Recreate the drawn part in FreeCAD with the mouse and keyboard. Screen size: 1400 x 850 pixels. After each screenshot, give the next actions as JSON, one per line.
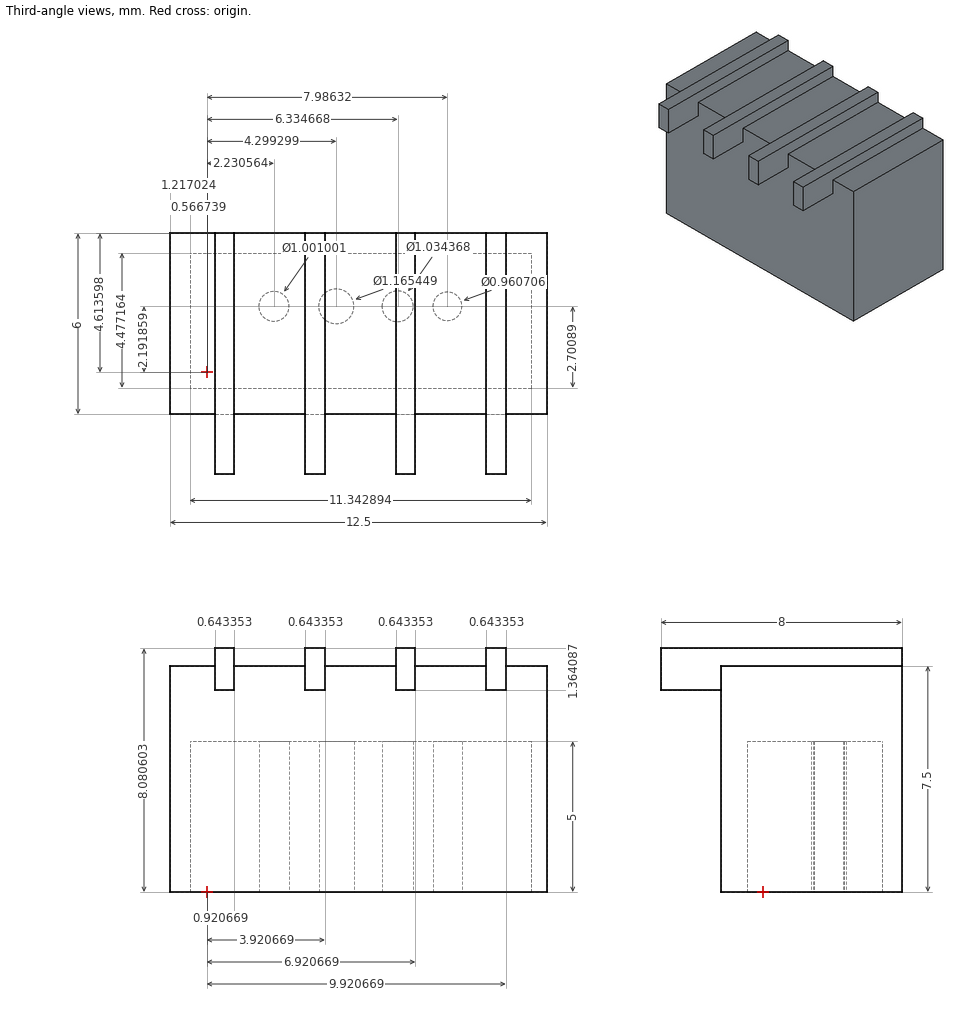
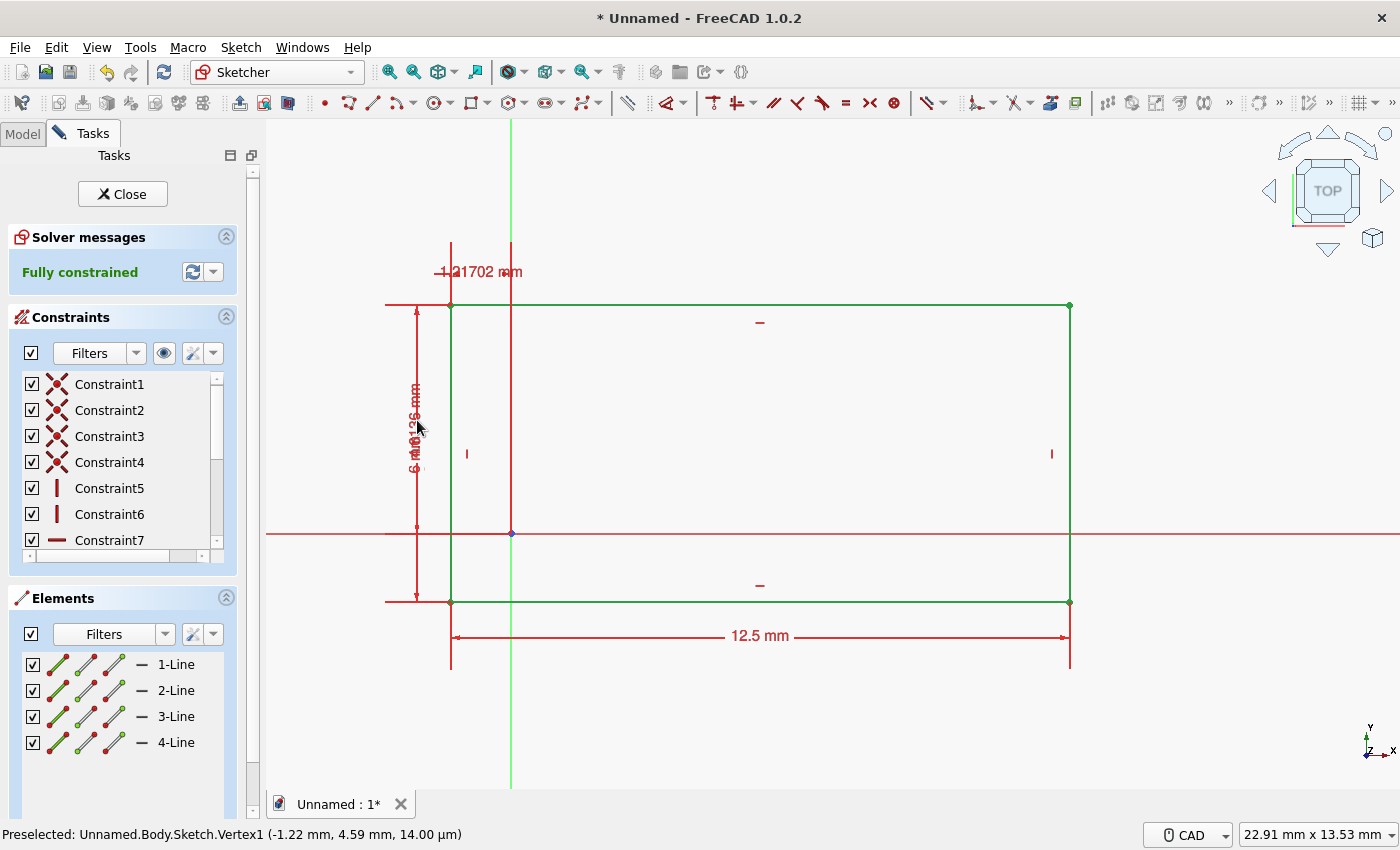
{"action": "left_click", "coordinate": [123, 194]}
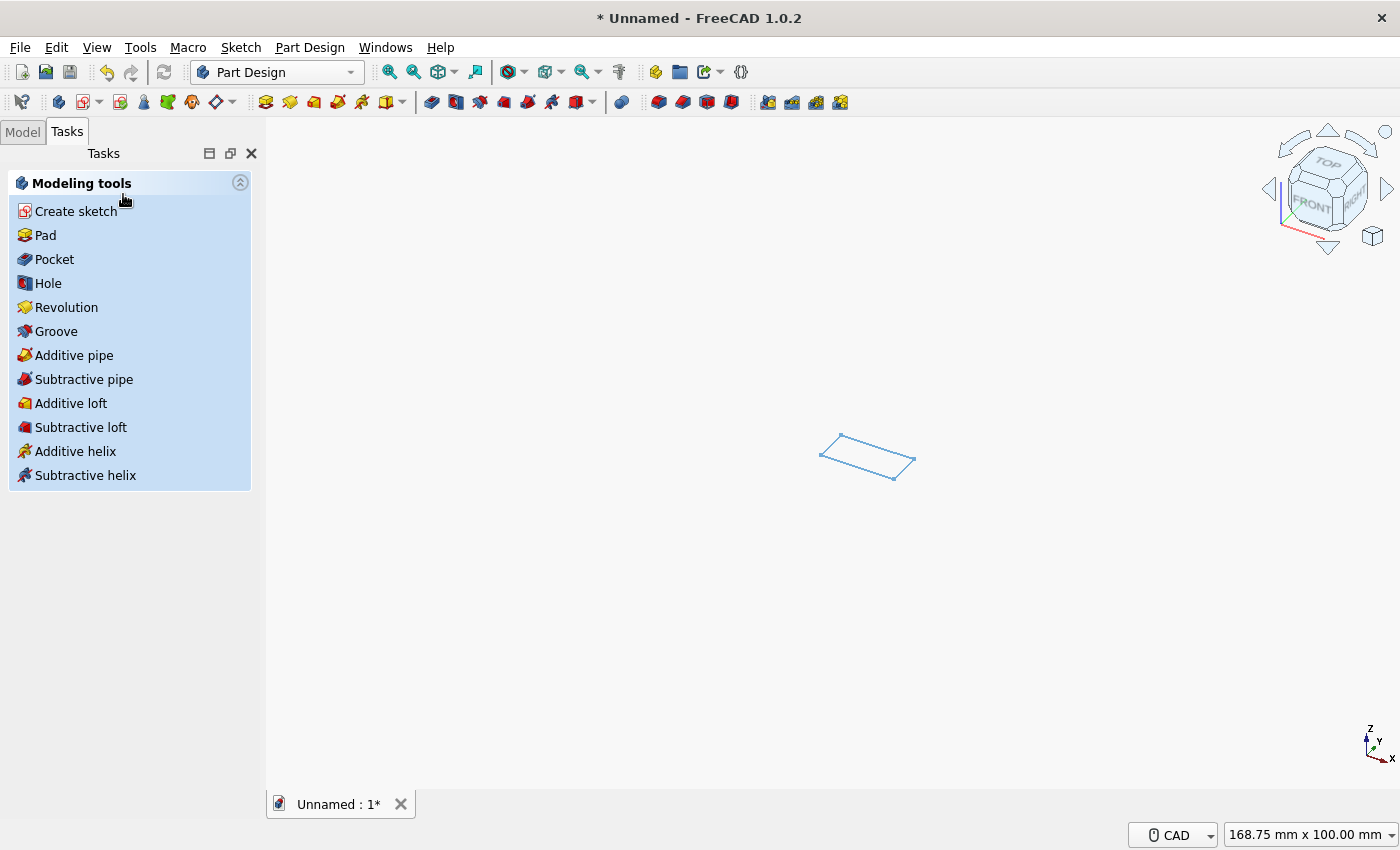
{"action": "left_click", "coordinate": [266, 102]}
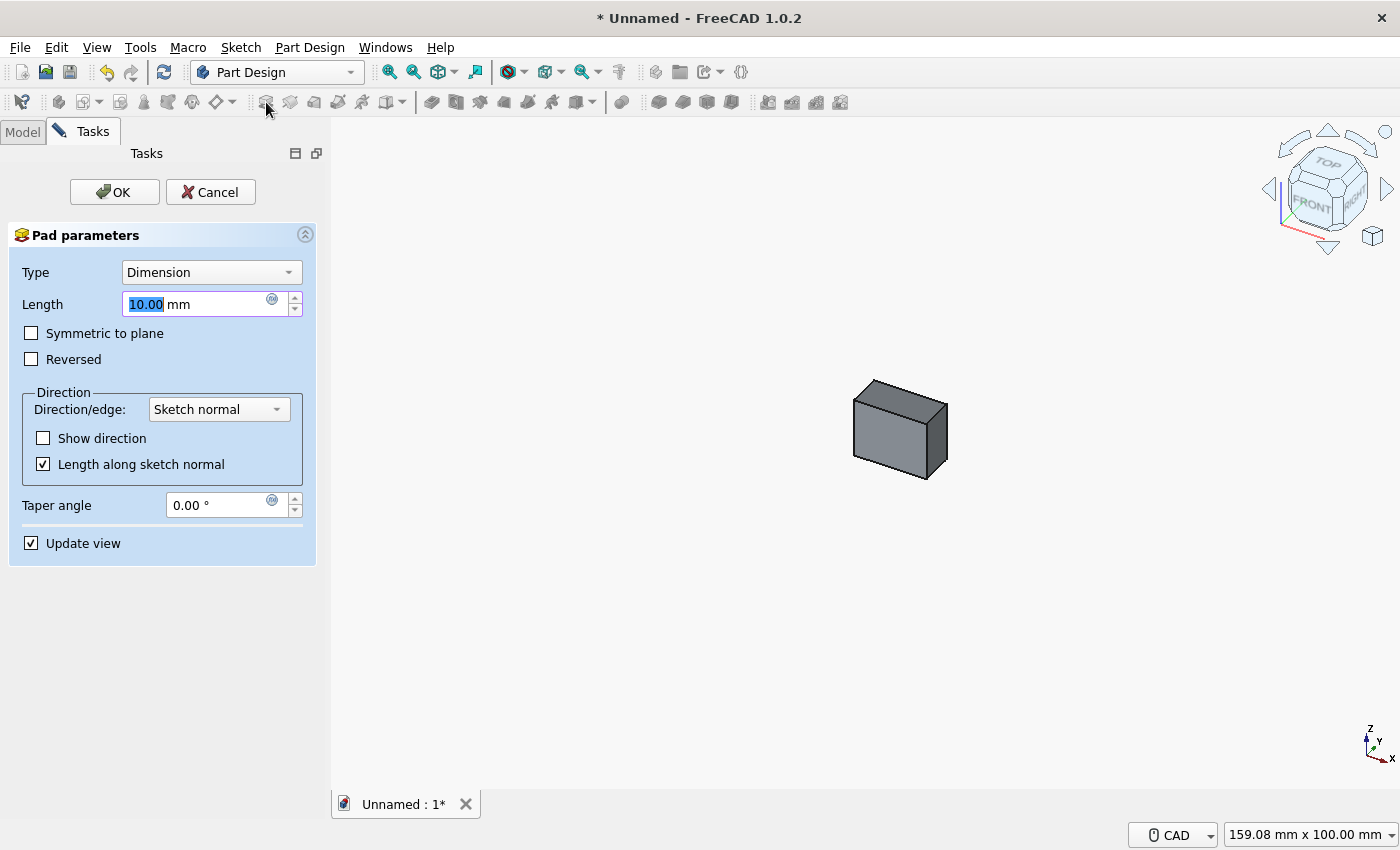
{"action": "type", "text": "7.5"}
{"action": "key", "text": "Tab"}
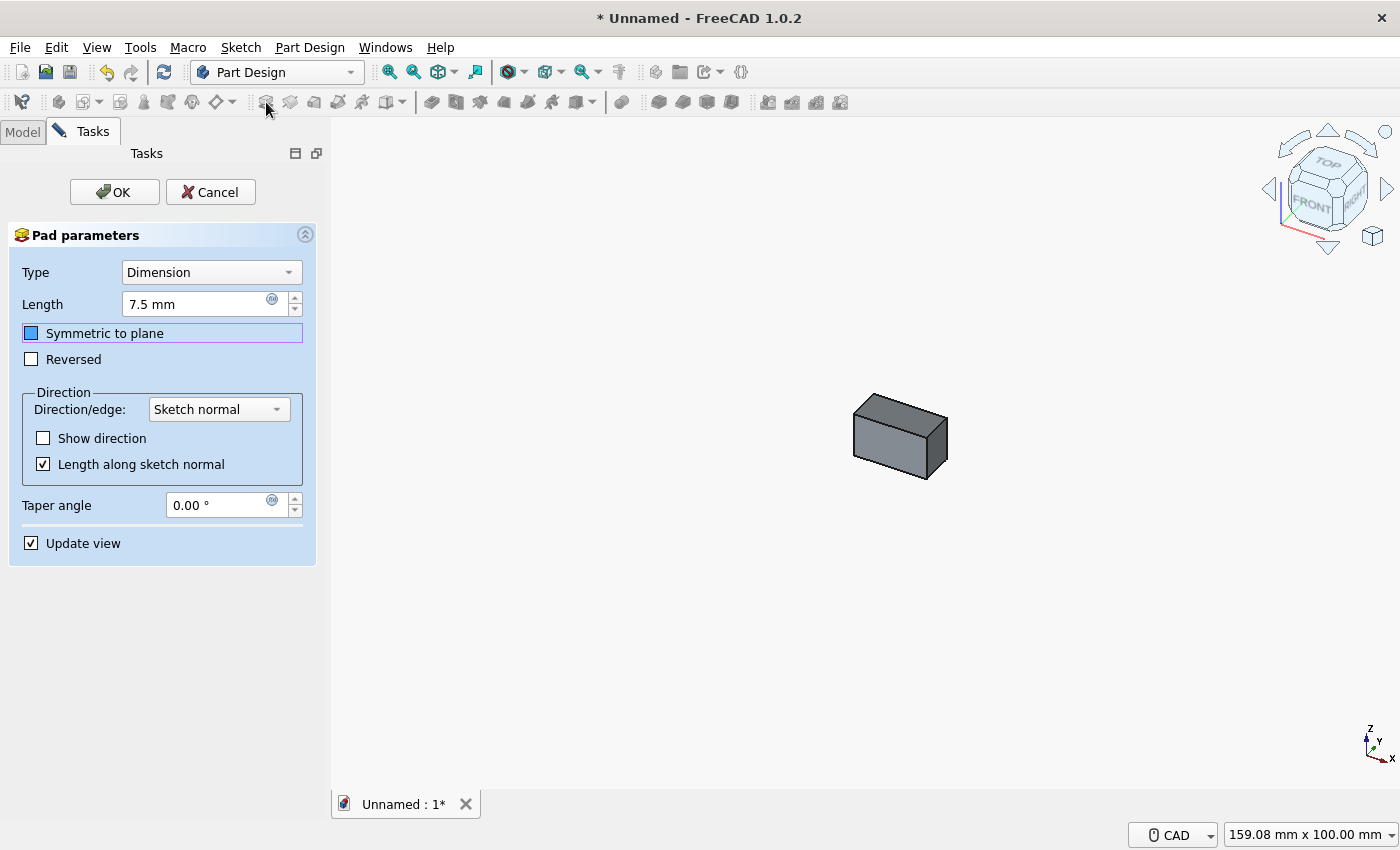
{"action": "left_click", "coordinate": [115, 192]}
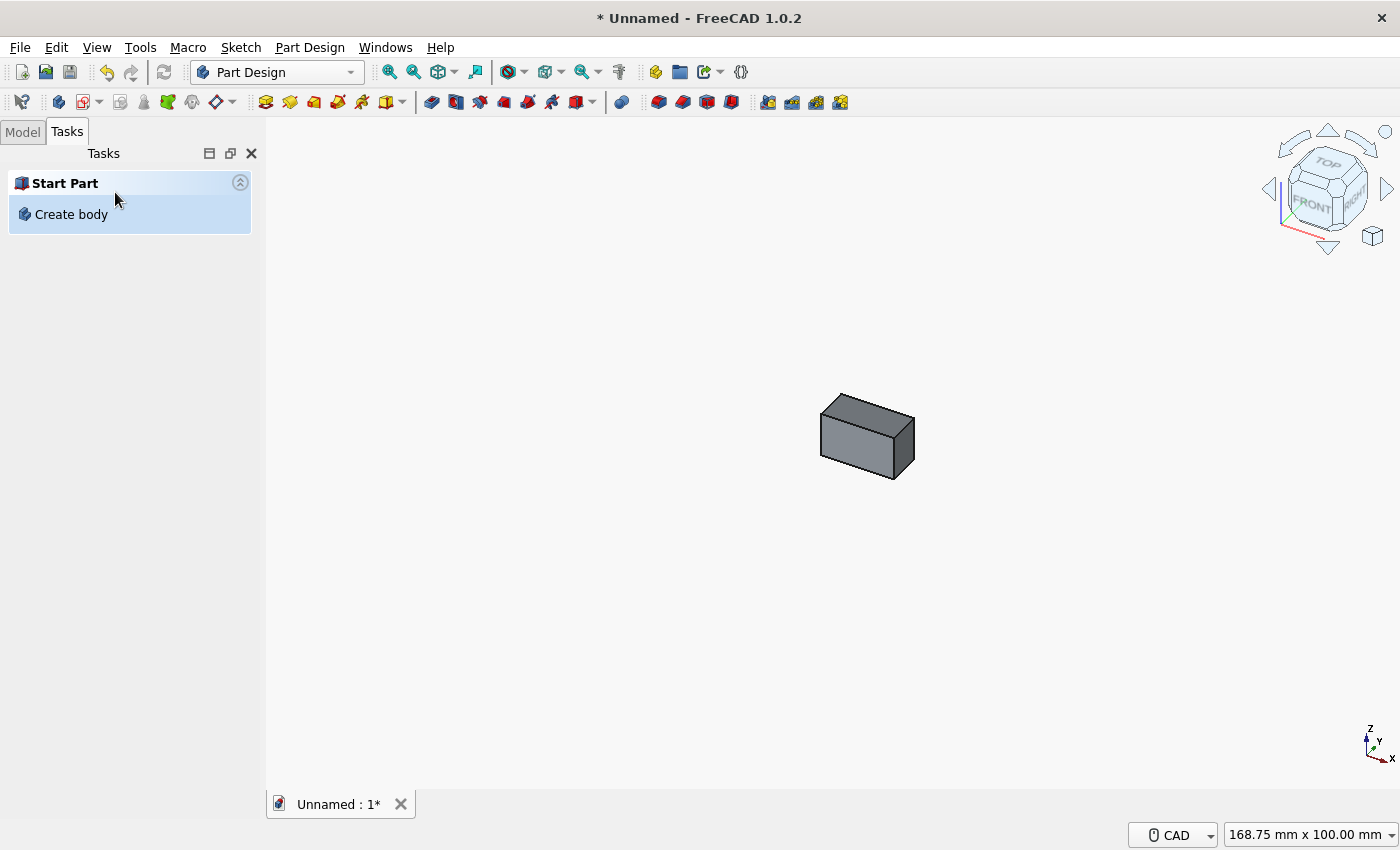
{"action": "key", "text": "v f"}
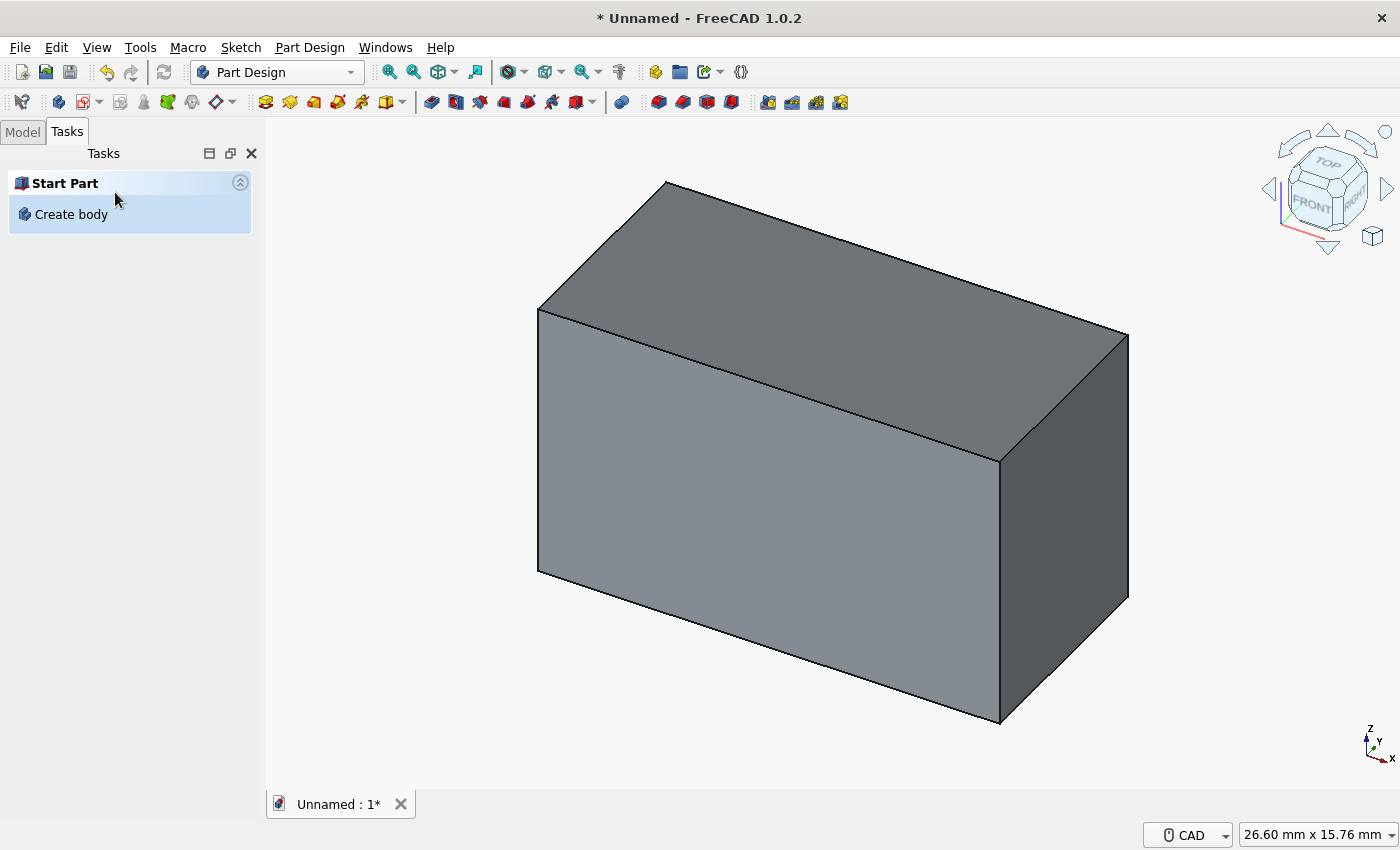
{"action": "left_click", "coordinate": [84, 102]}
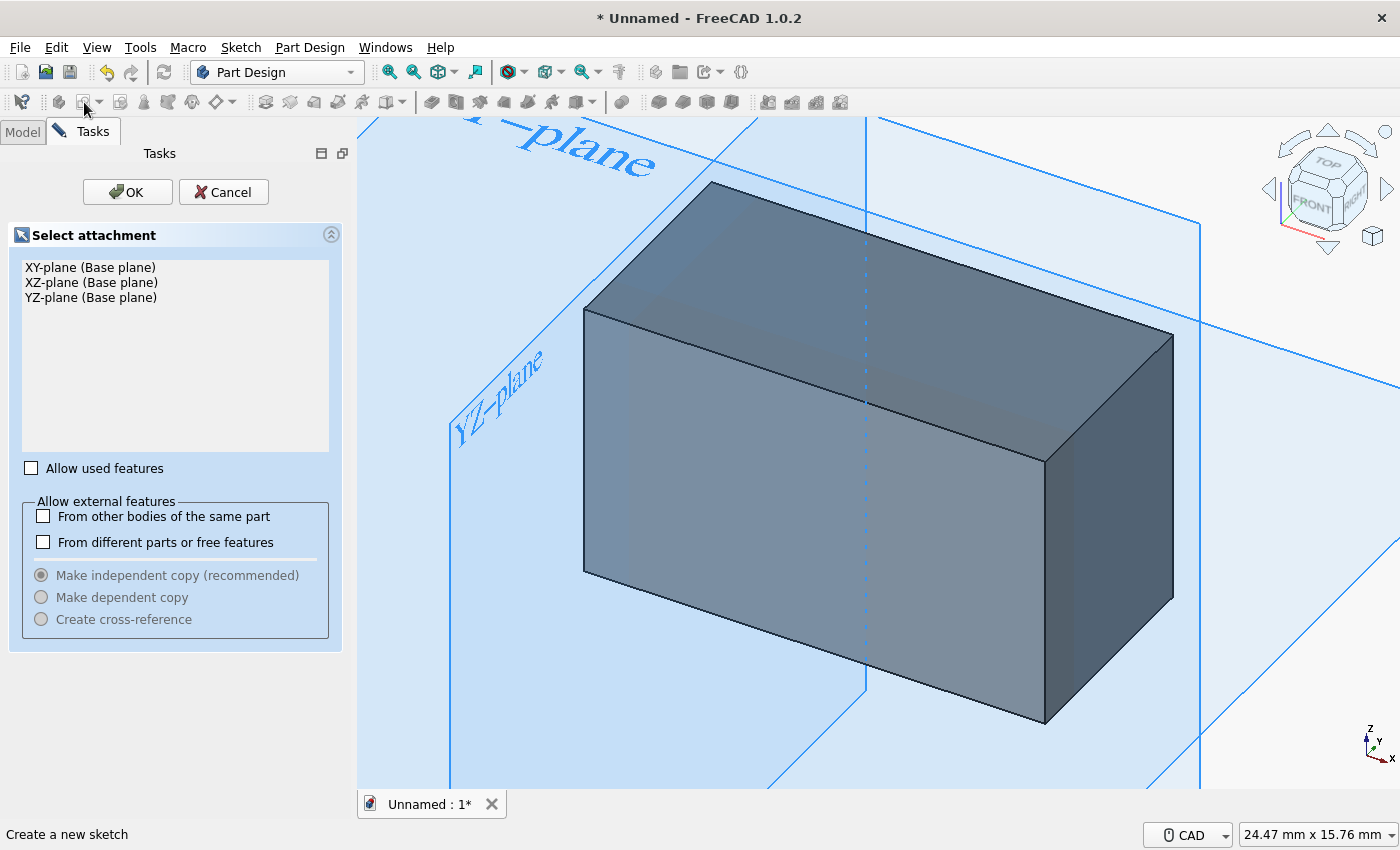
{"action": "left_click", "coordinate": [82, 268]}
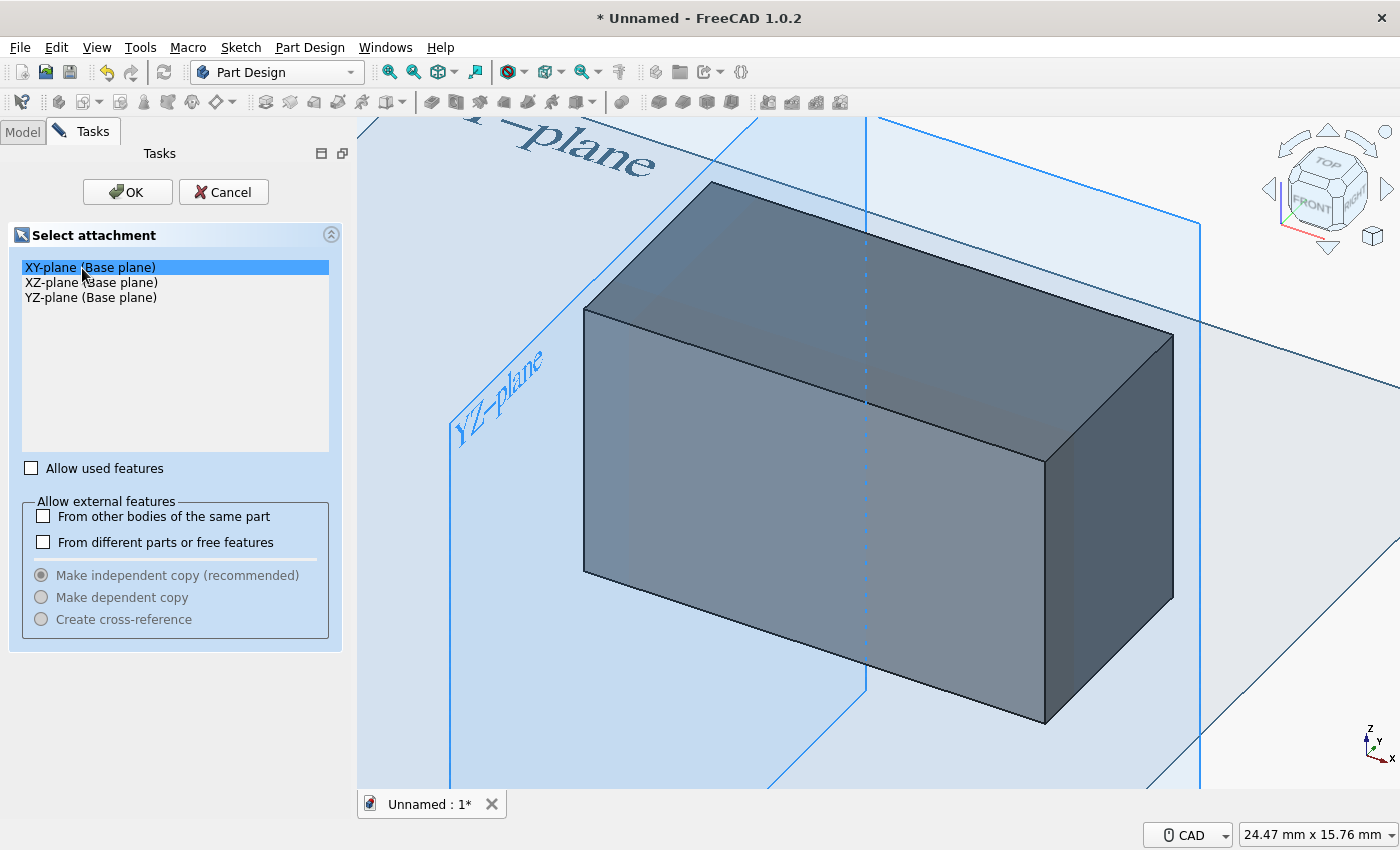
{"action": "left_click", "coordinate": [128, 192]}